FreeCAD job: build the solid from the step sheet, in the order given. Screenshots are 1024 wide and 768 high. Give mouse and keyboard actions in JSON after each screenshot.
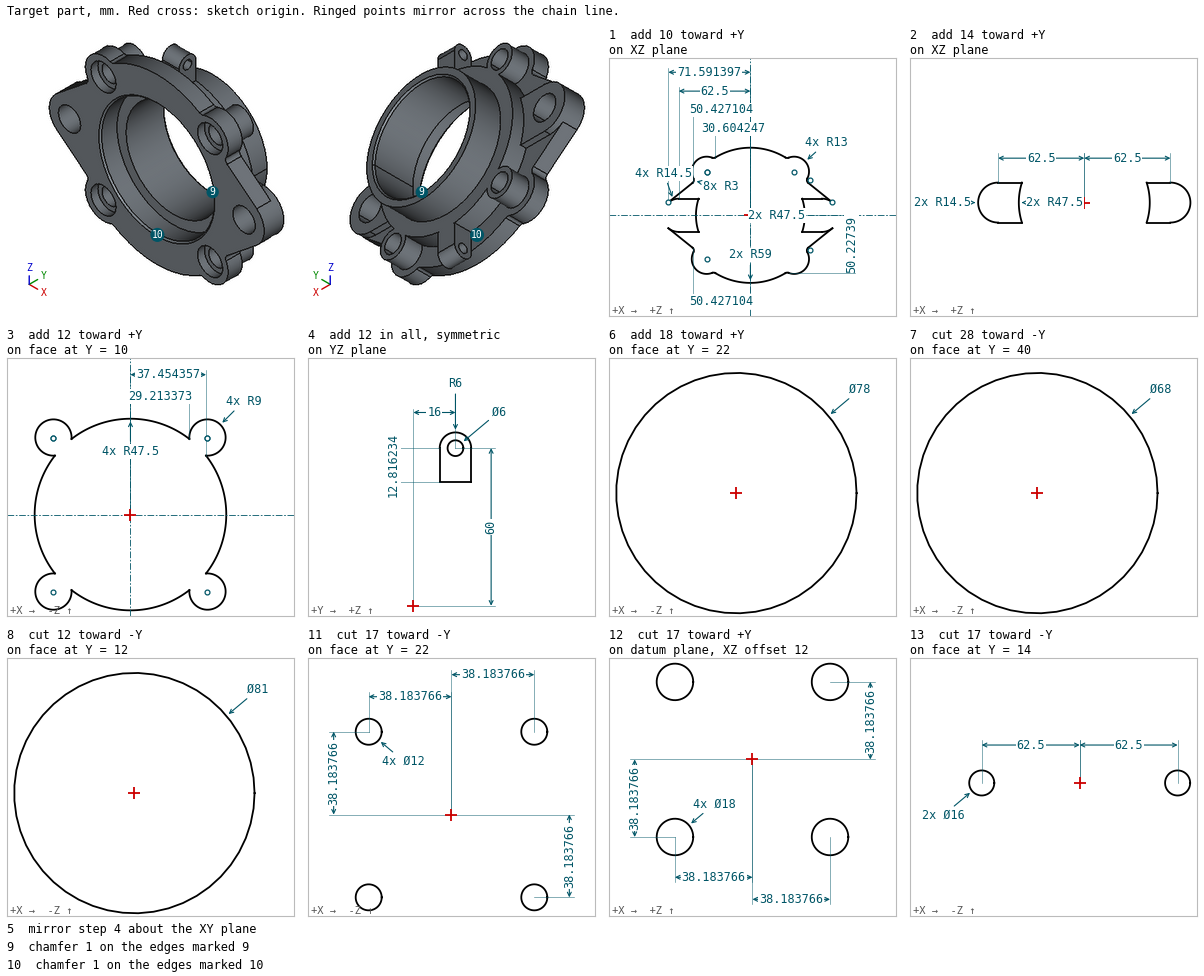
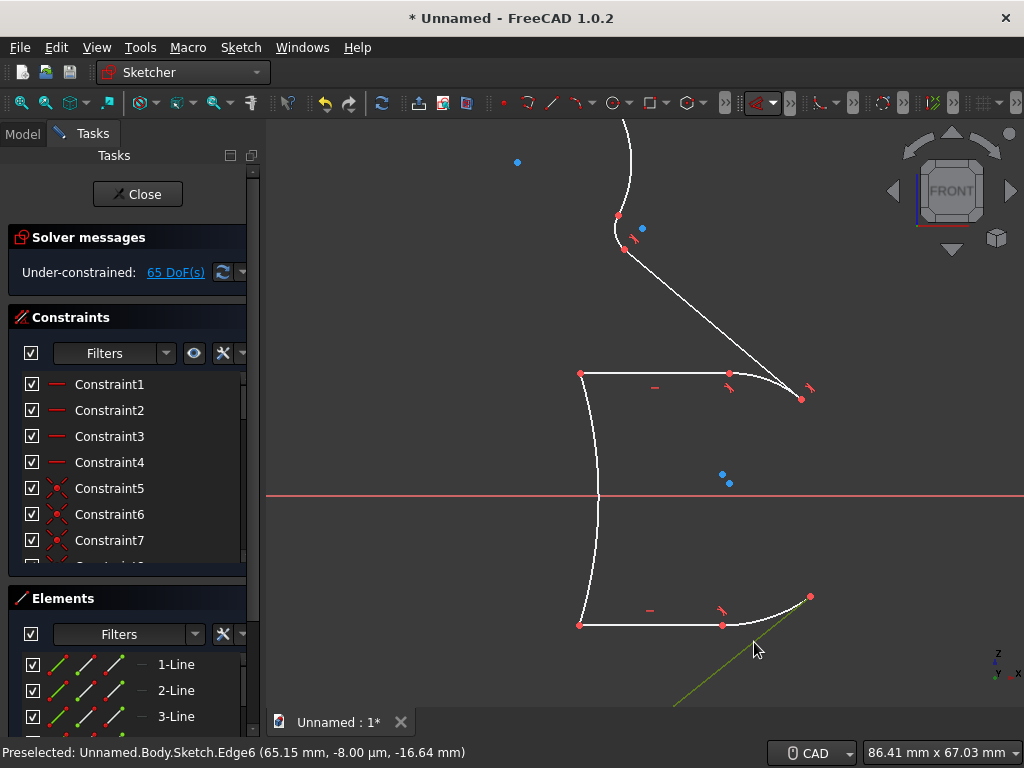
{"action": "left_click", "coordinate": [750, 623]}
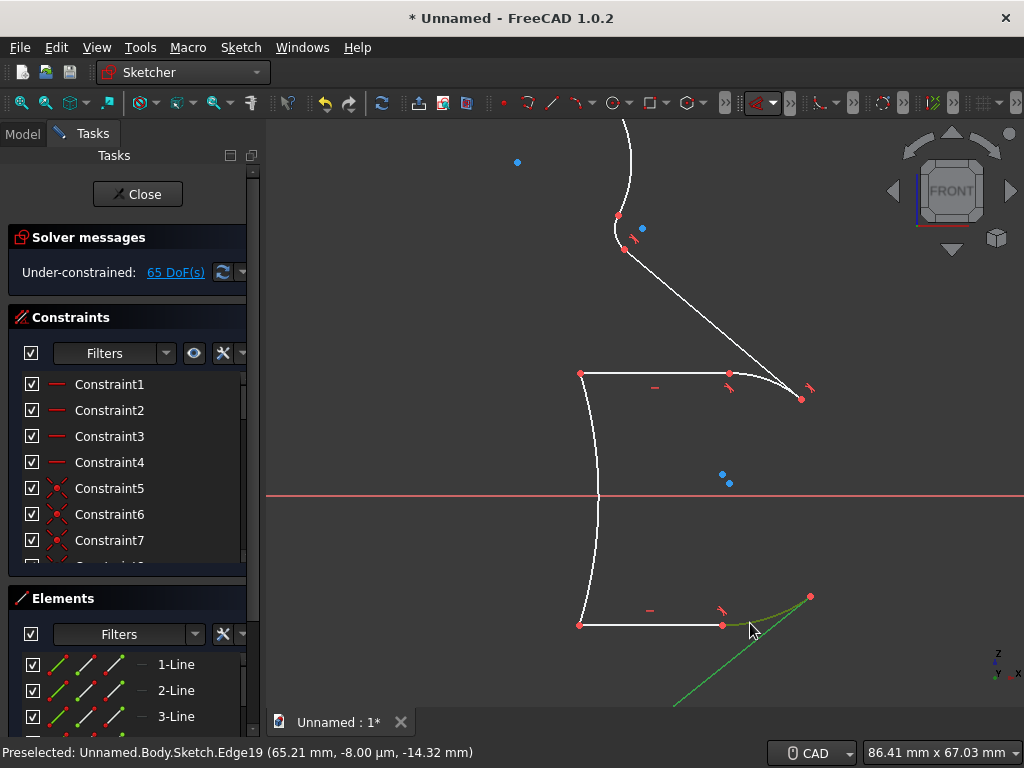
{"action": "key", "text": "t"}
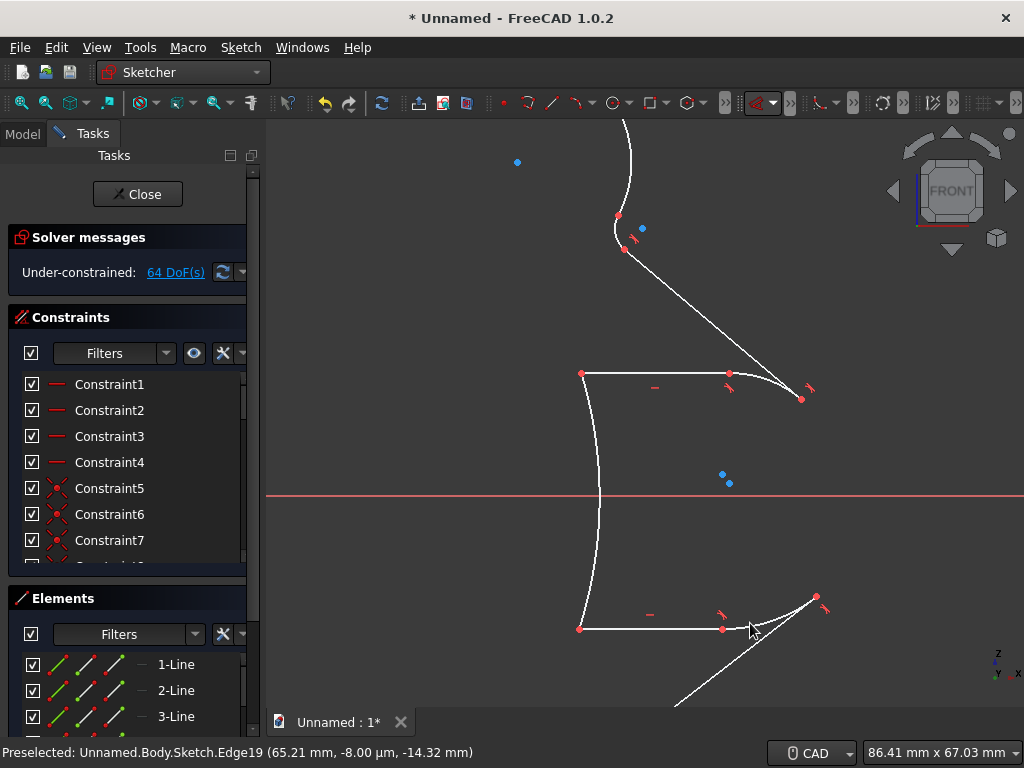
{"action": "left_click", "coordinate": [759, 642]}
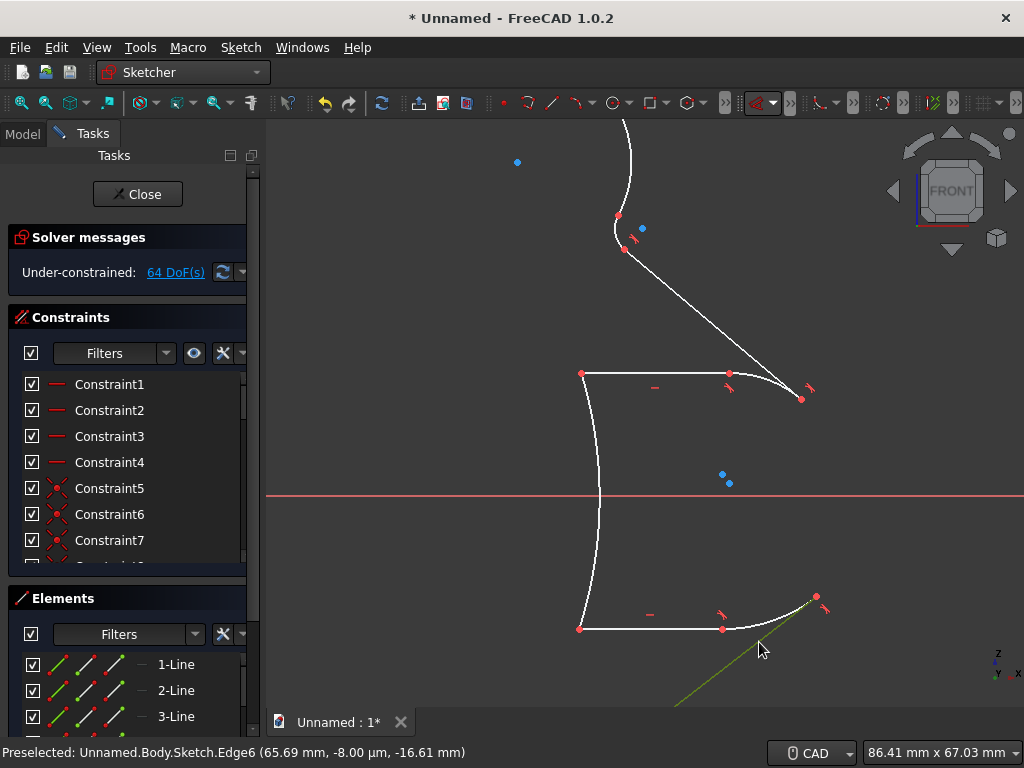
{"action": "scroll", "coordinate": [747, 377], "scroll_direction": "down", "scroll_amount": 6}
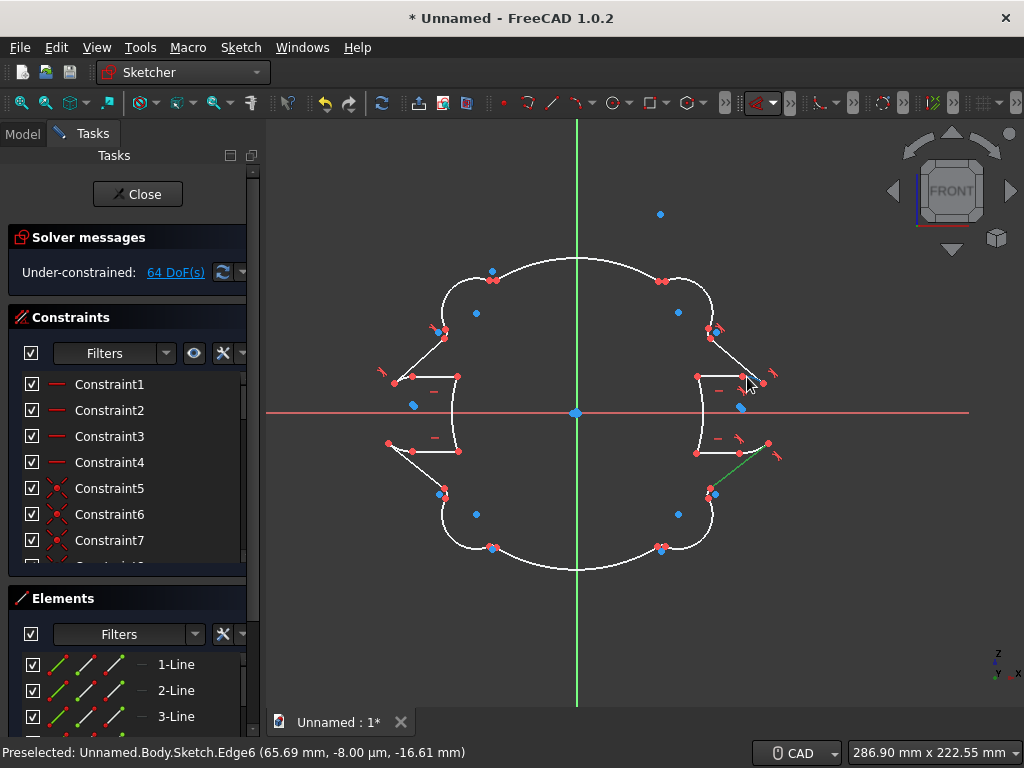
{"action": "scroll", "coordinate": [708, 491], "scroll_direction": "up", "scroll_amount": 8}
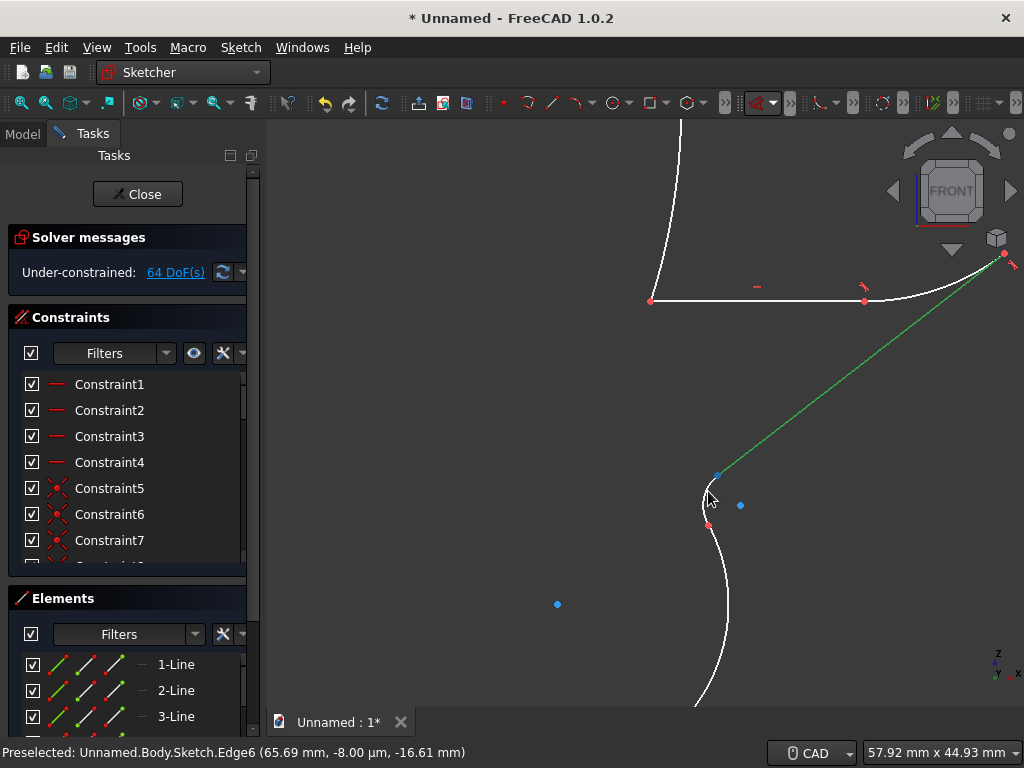
{"action": "left_click", "coordinate": [707, 489]}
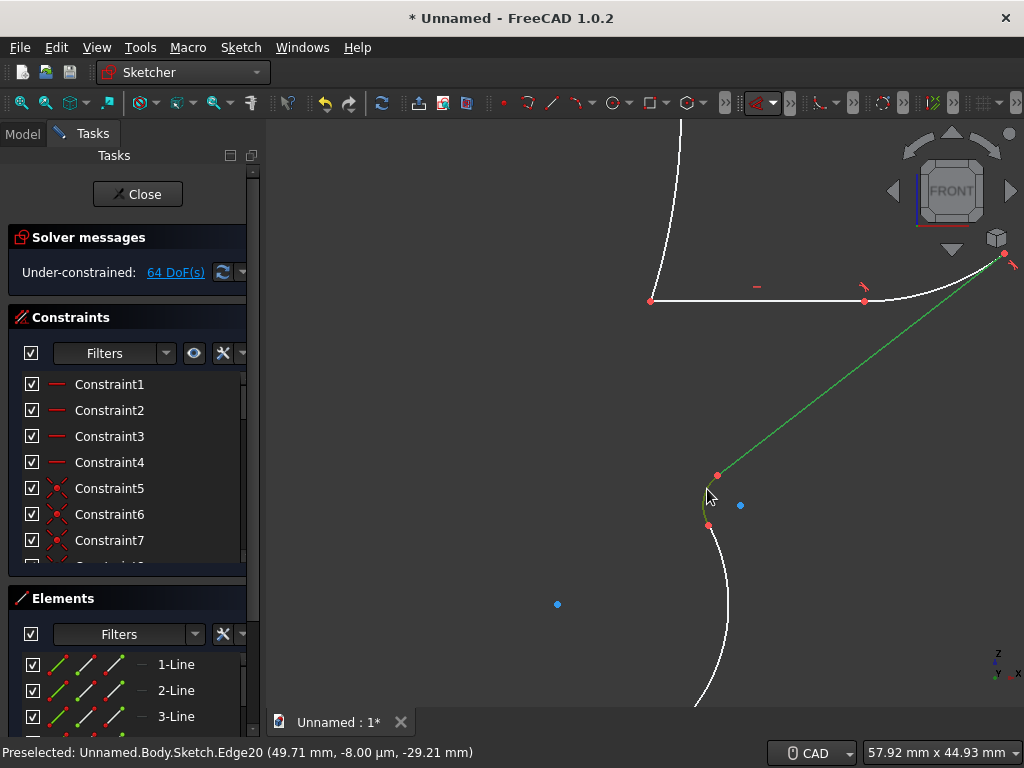
{"action": "key", "text": "t"}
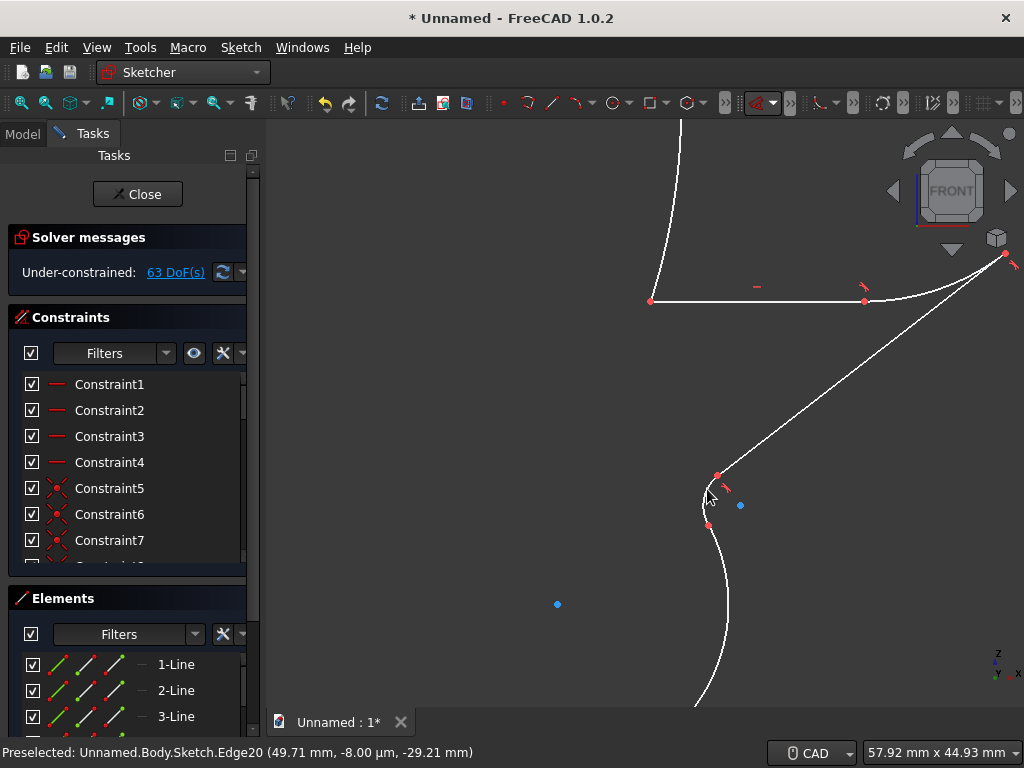
{"action": "scroll", "coordinate": [708, 491], "scroll_direction": "down", "scroll_amount": 8}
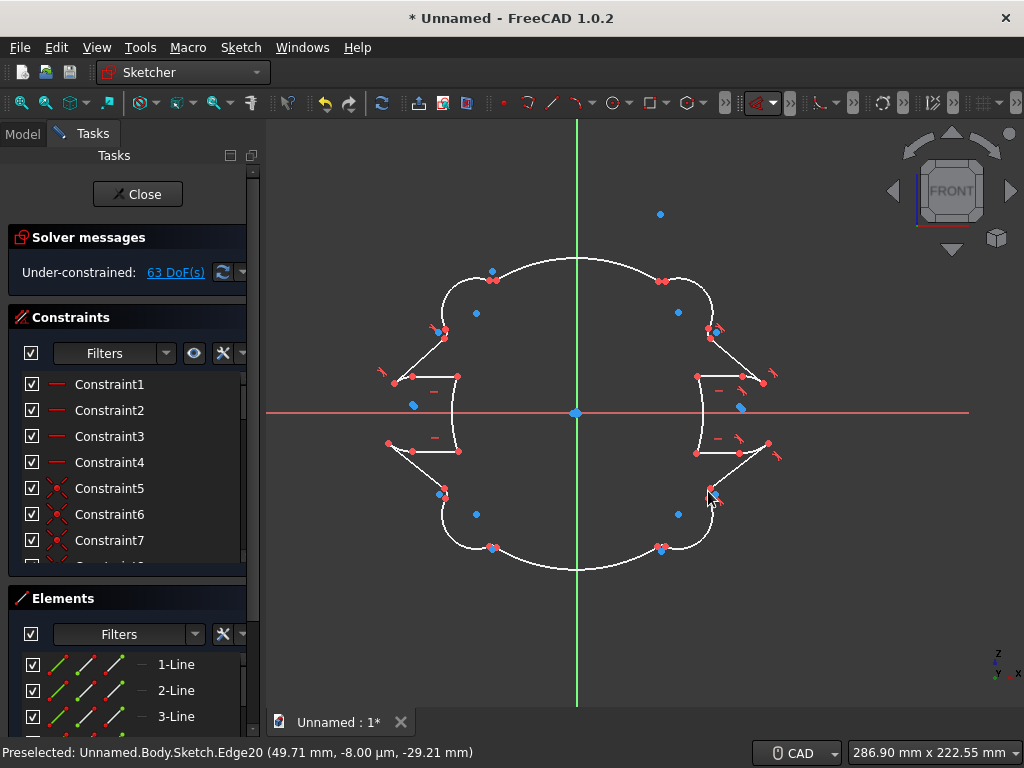
{"action": "left_click", "coordinate": [428, 475]}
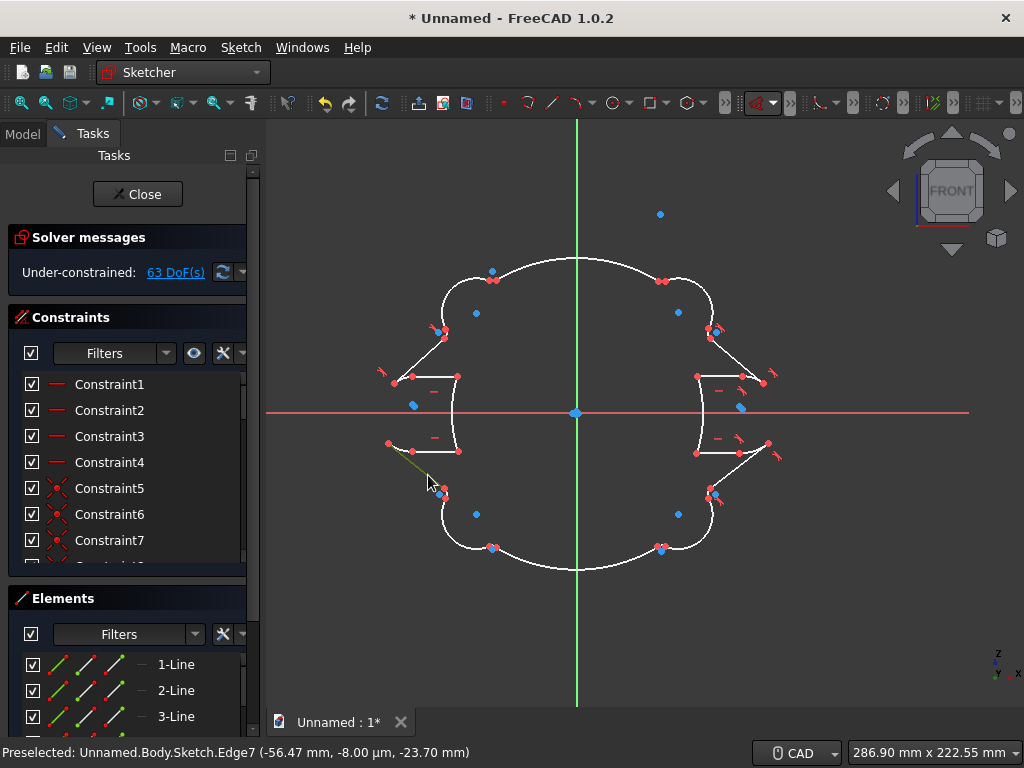
{"action": "scroll", "coordinate": [447, 493], "scroll_direction": "up", "scroll_amount": 5}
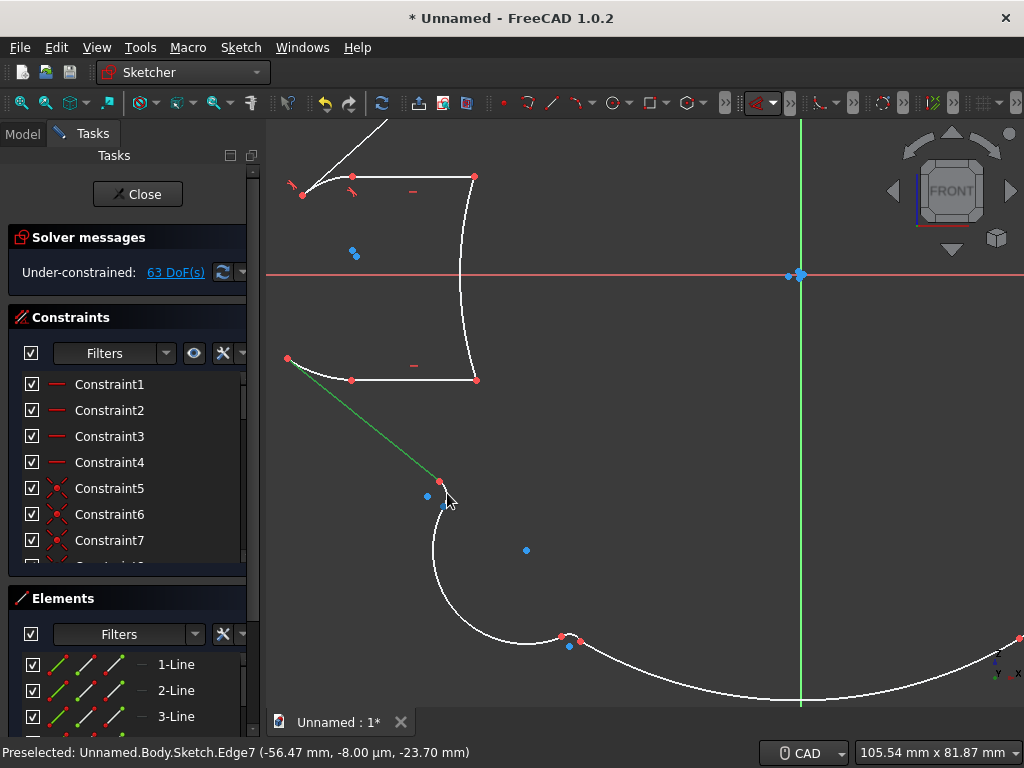
{"action": "left_click", "coordinate": [447, 493]}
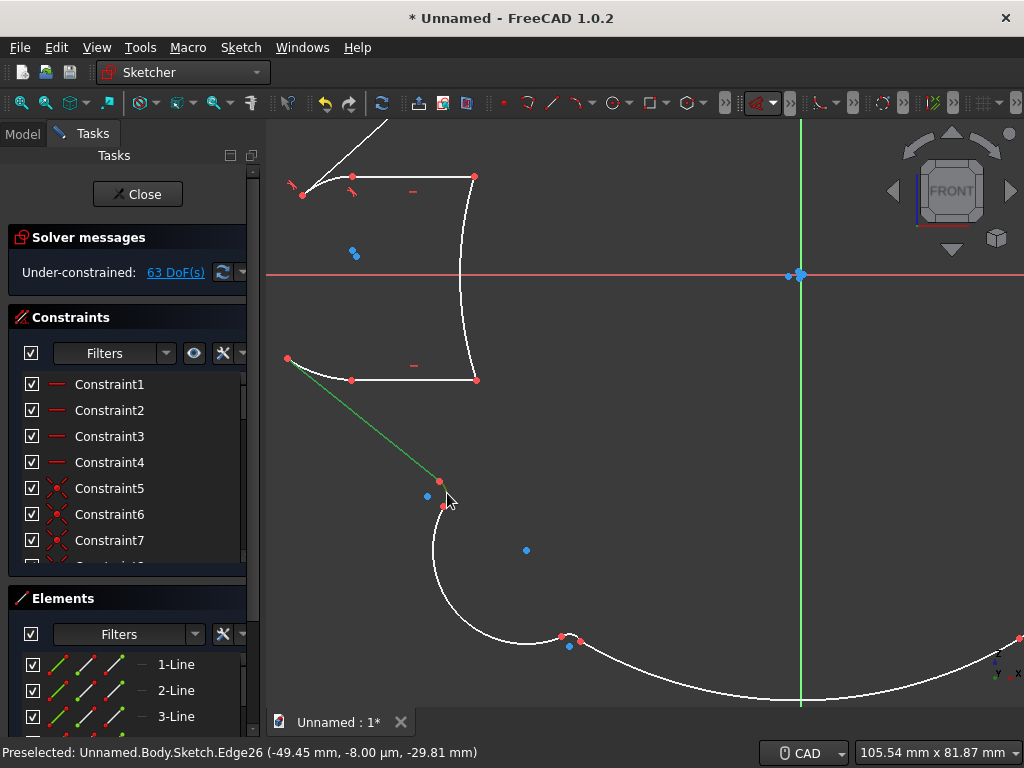
{"action": "key", "text": "t"}